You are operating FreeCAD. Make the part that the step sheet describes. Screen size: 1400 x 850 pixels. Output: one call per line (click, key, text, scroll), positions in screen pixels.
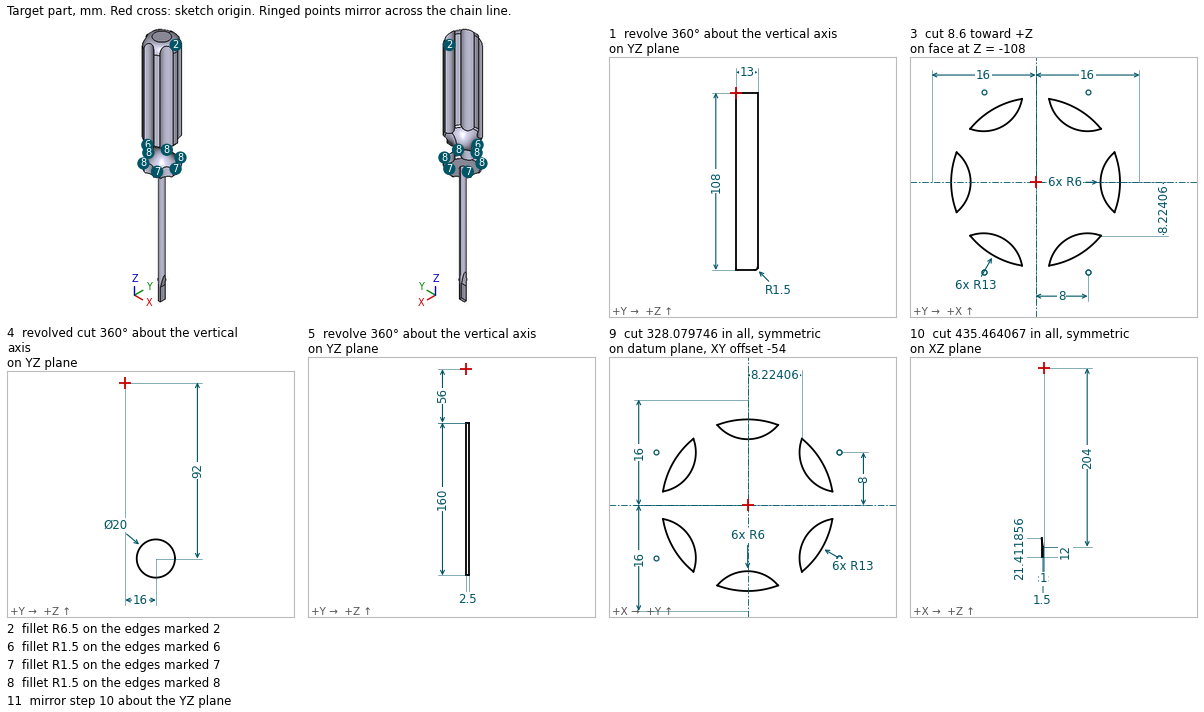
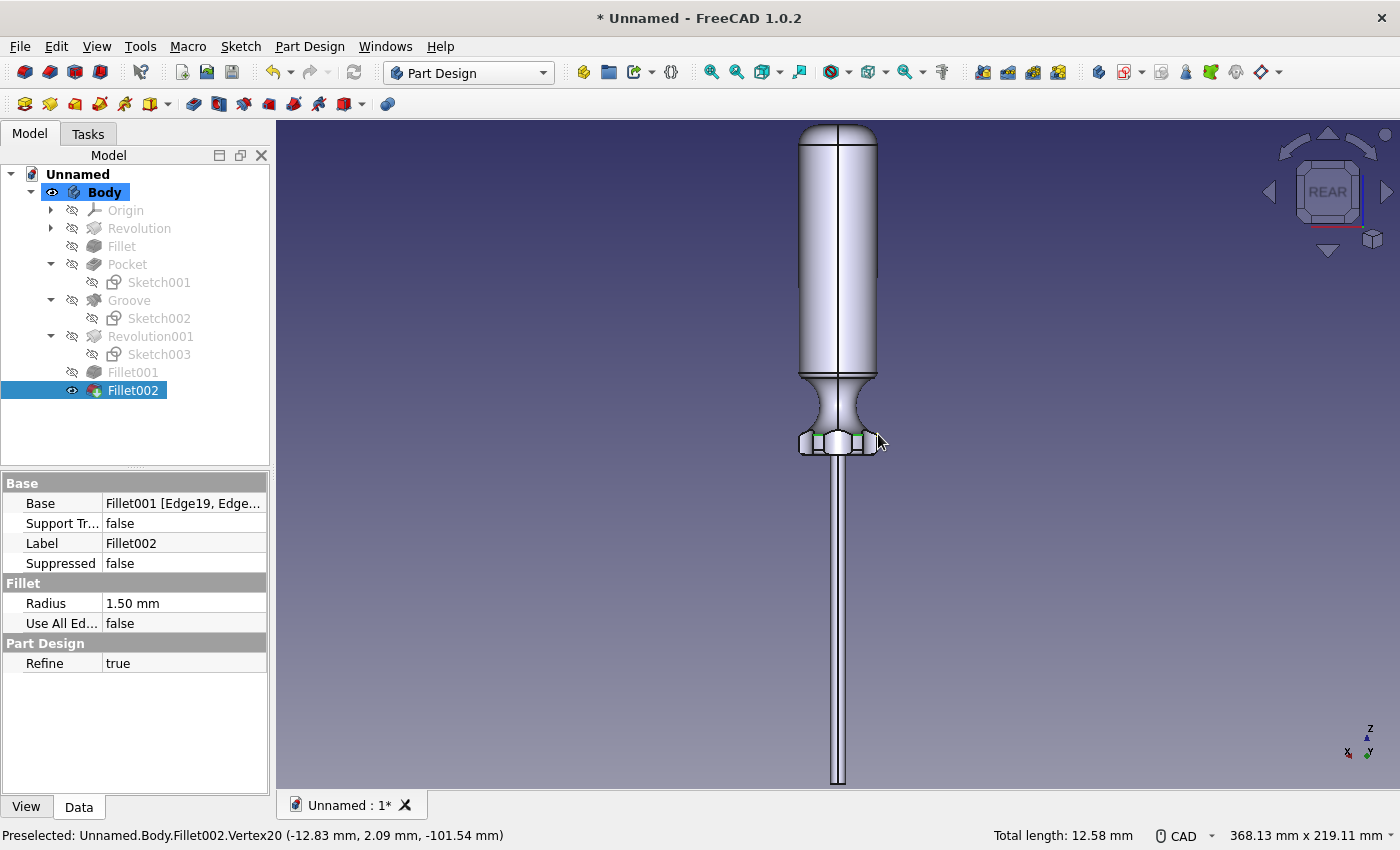
key(6)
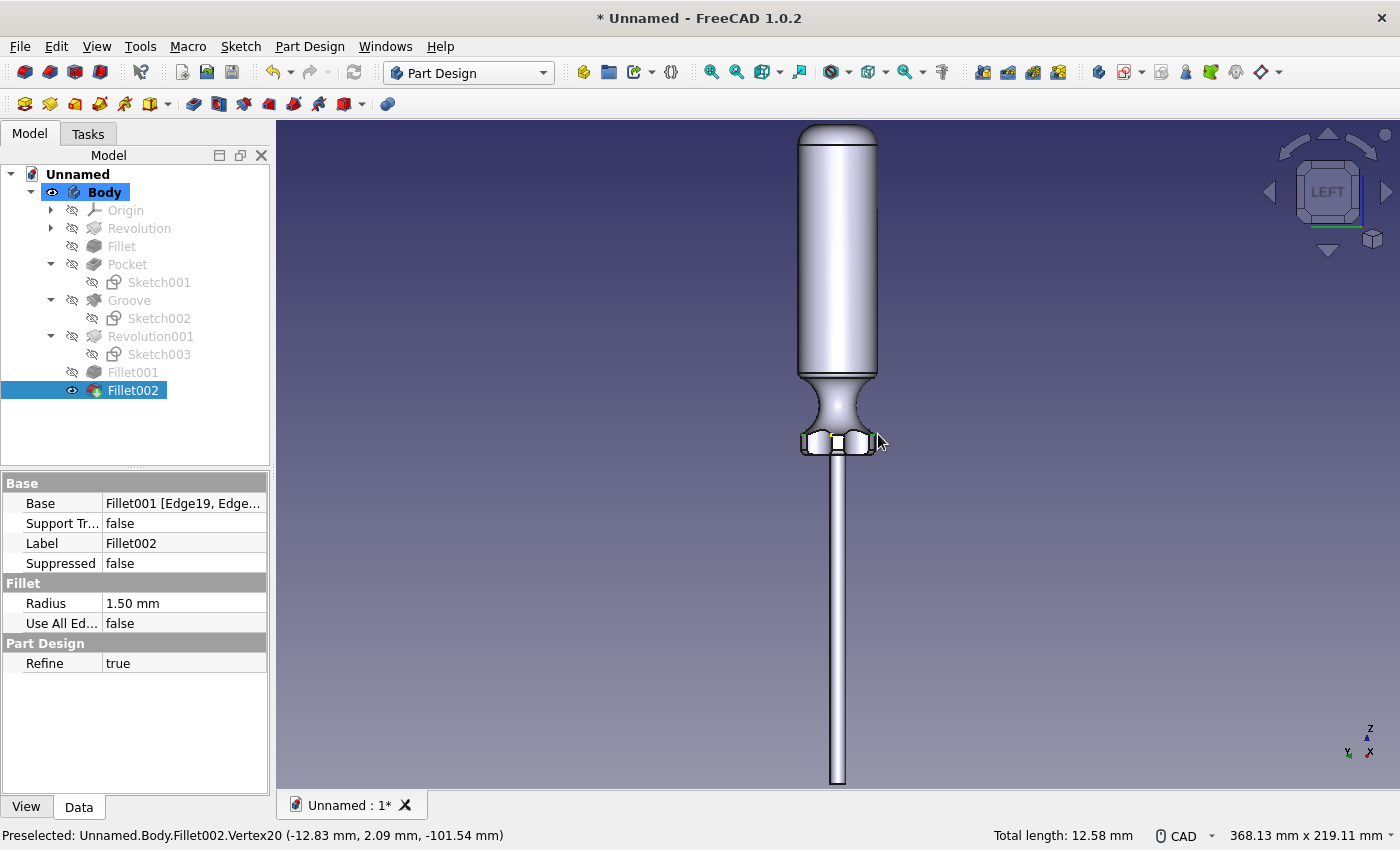
click(838, 434, ctrl)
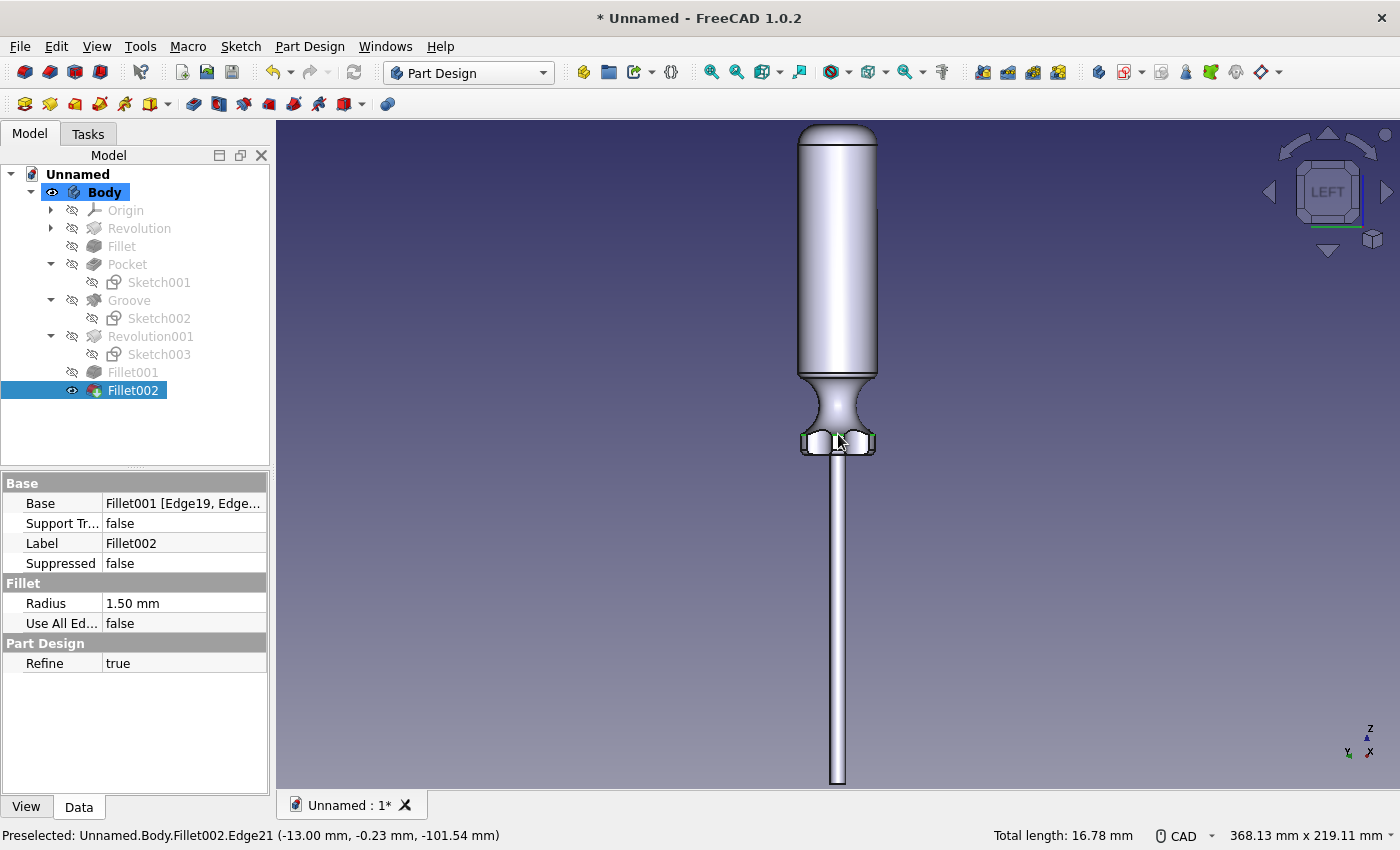
click(25, 72)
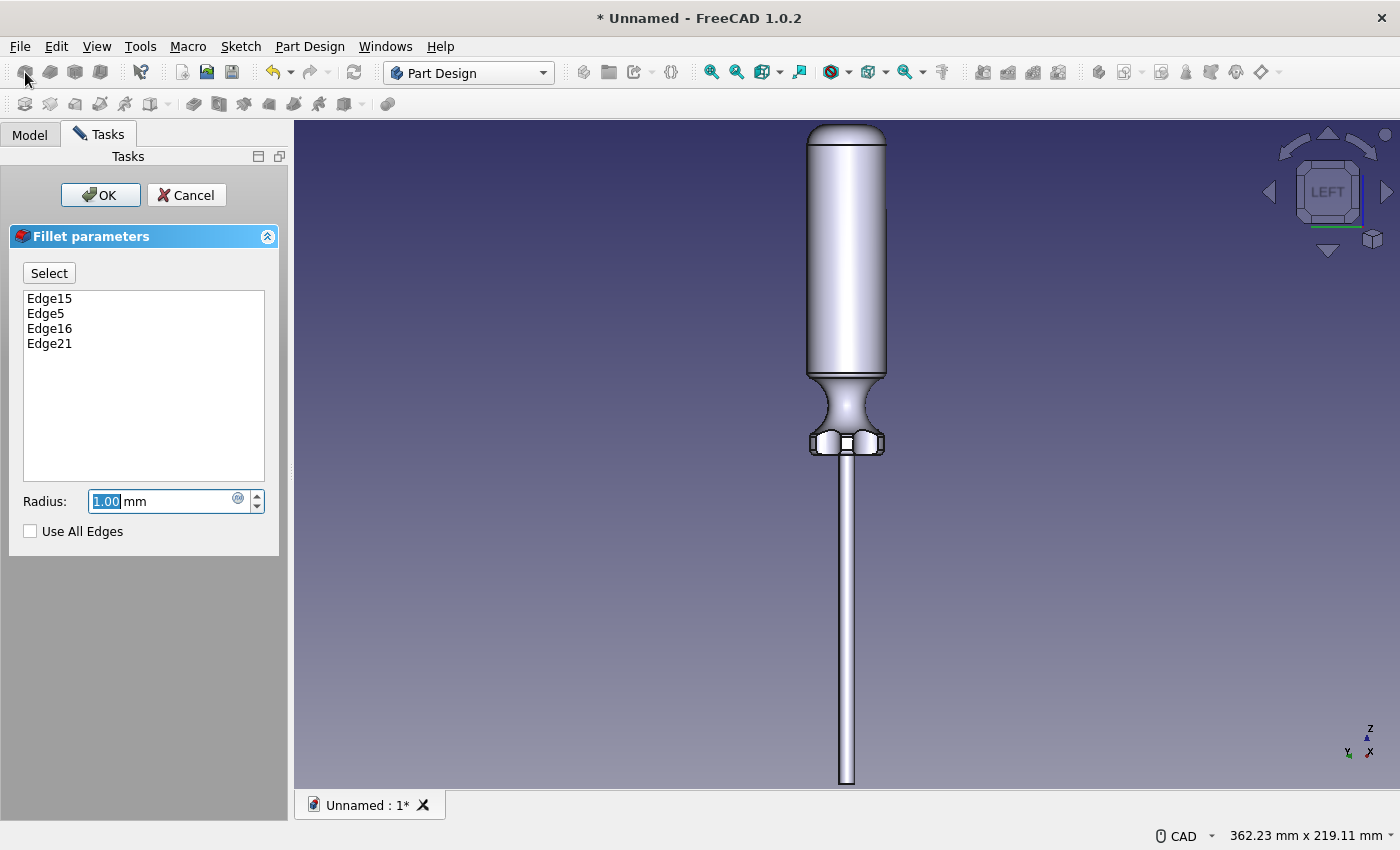
text(1.5)
key(Tab)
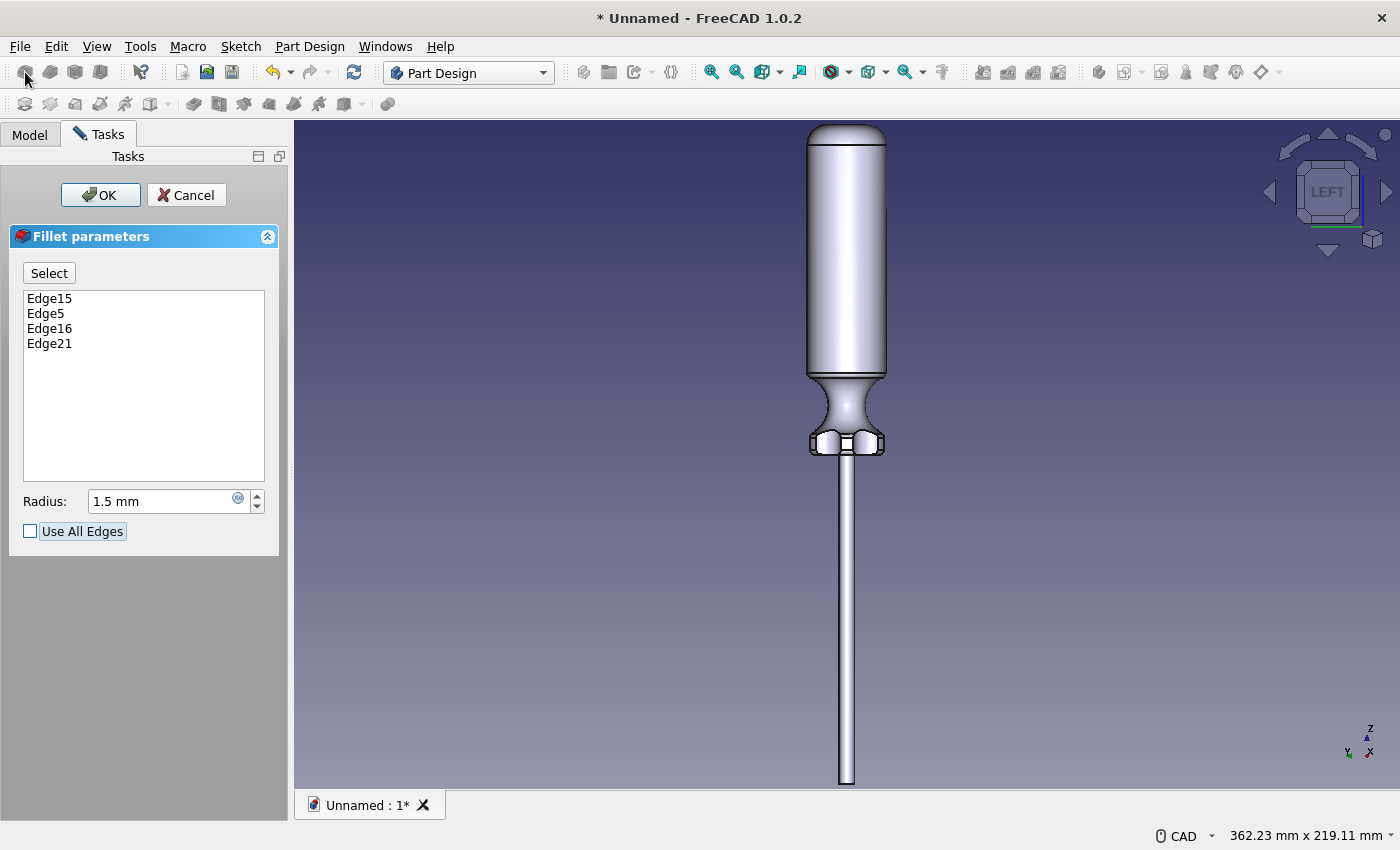
click(101, 195)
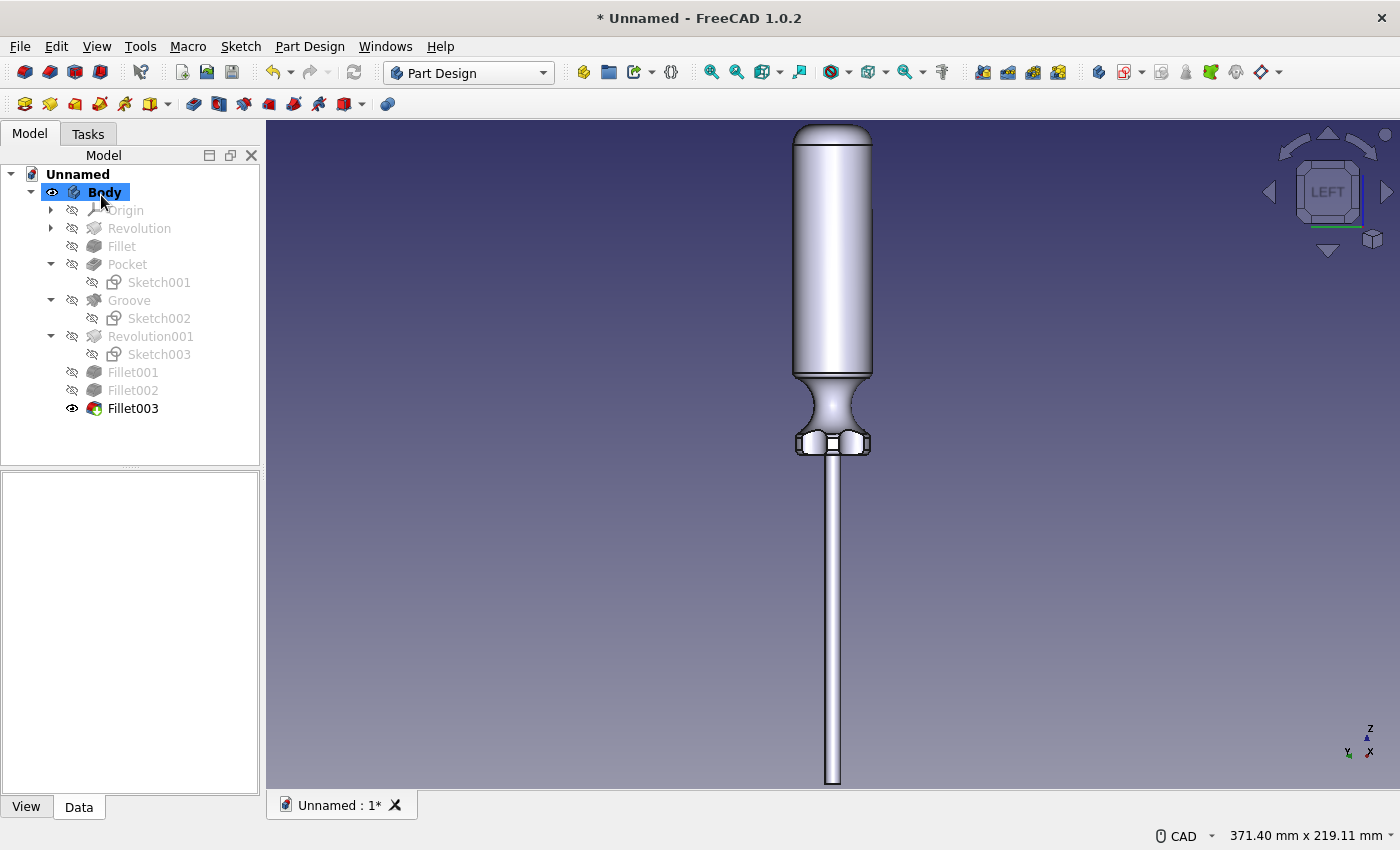
click(51, 210)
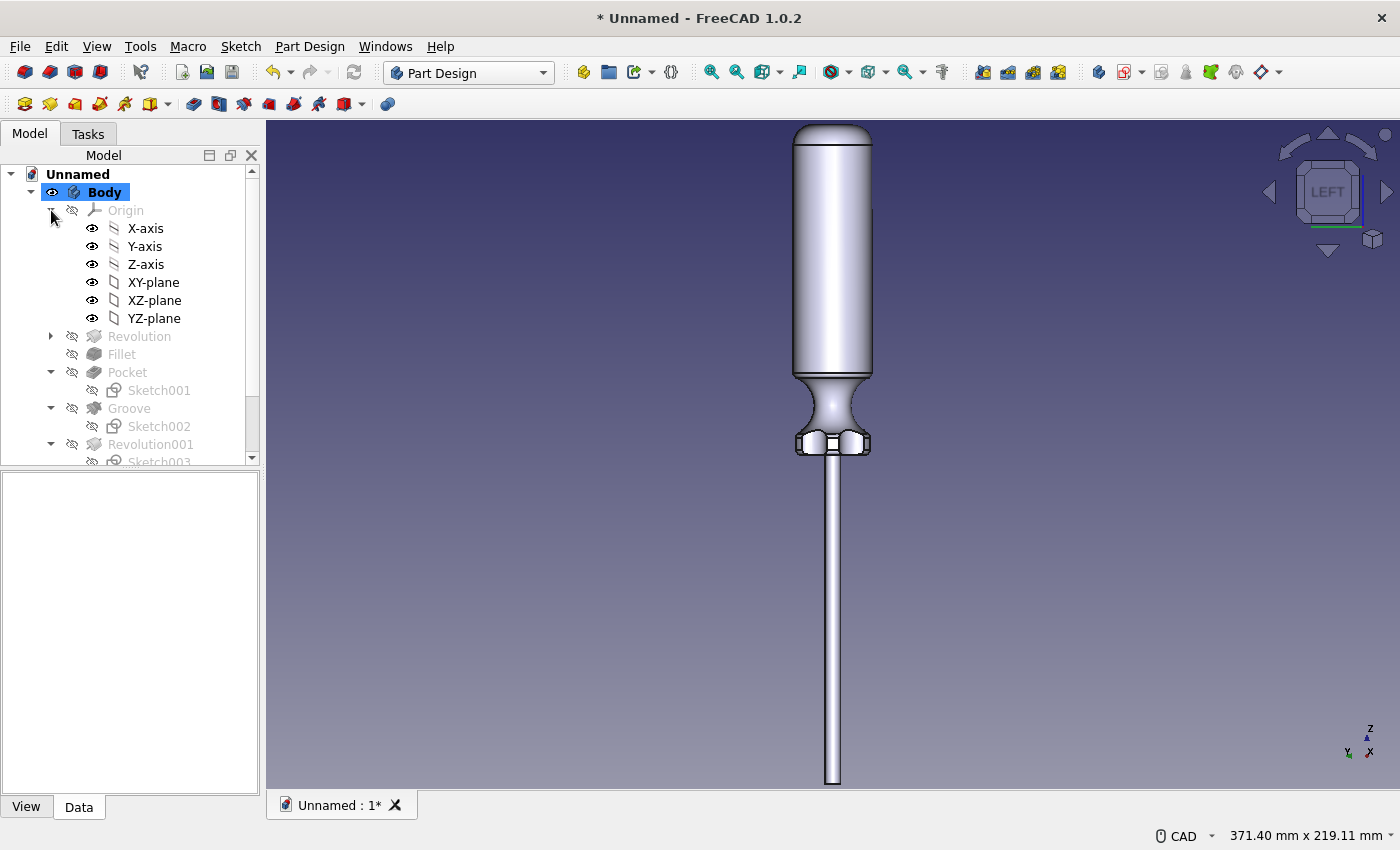
click(137, 282)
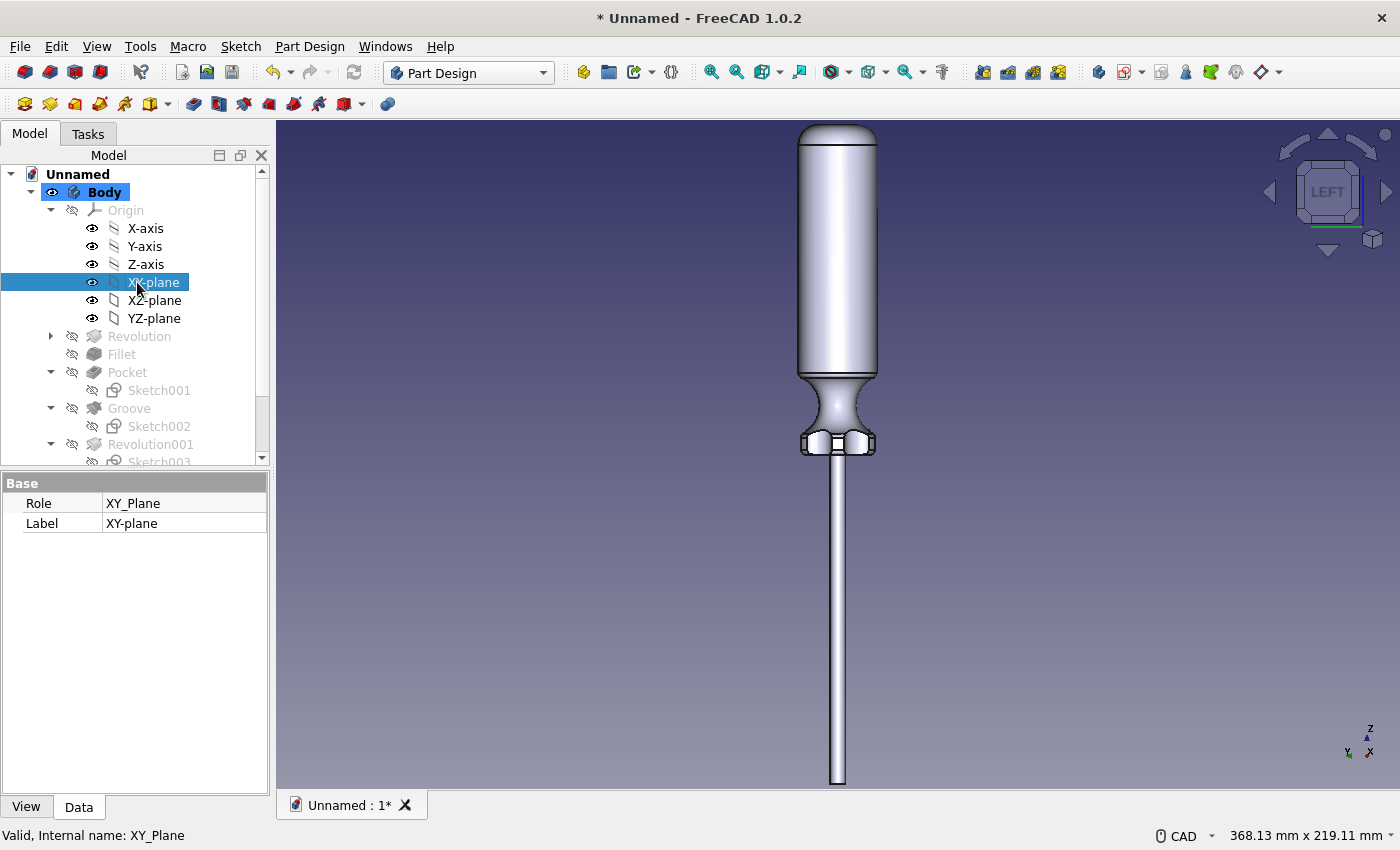
click(1260, 72)